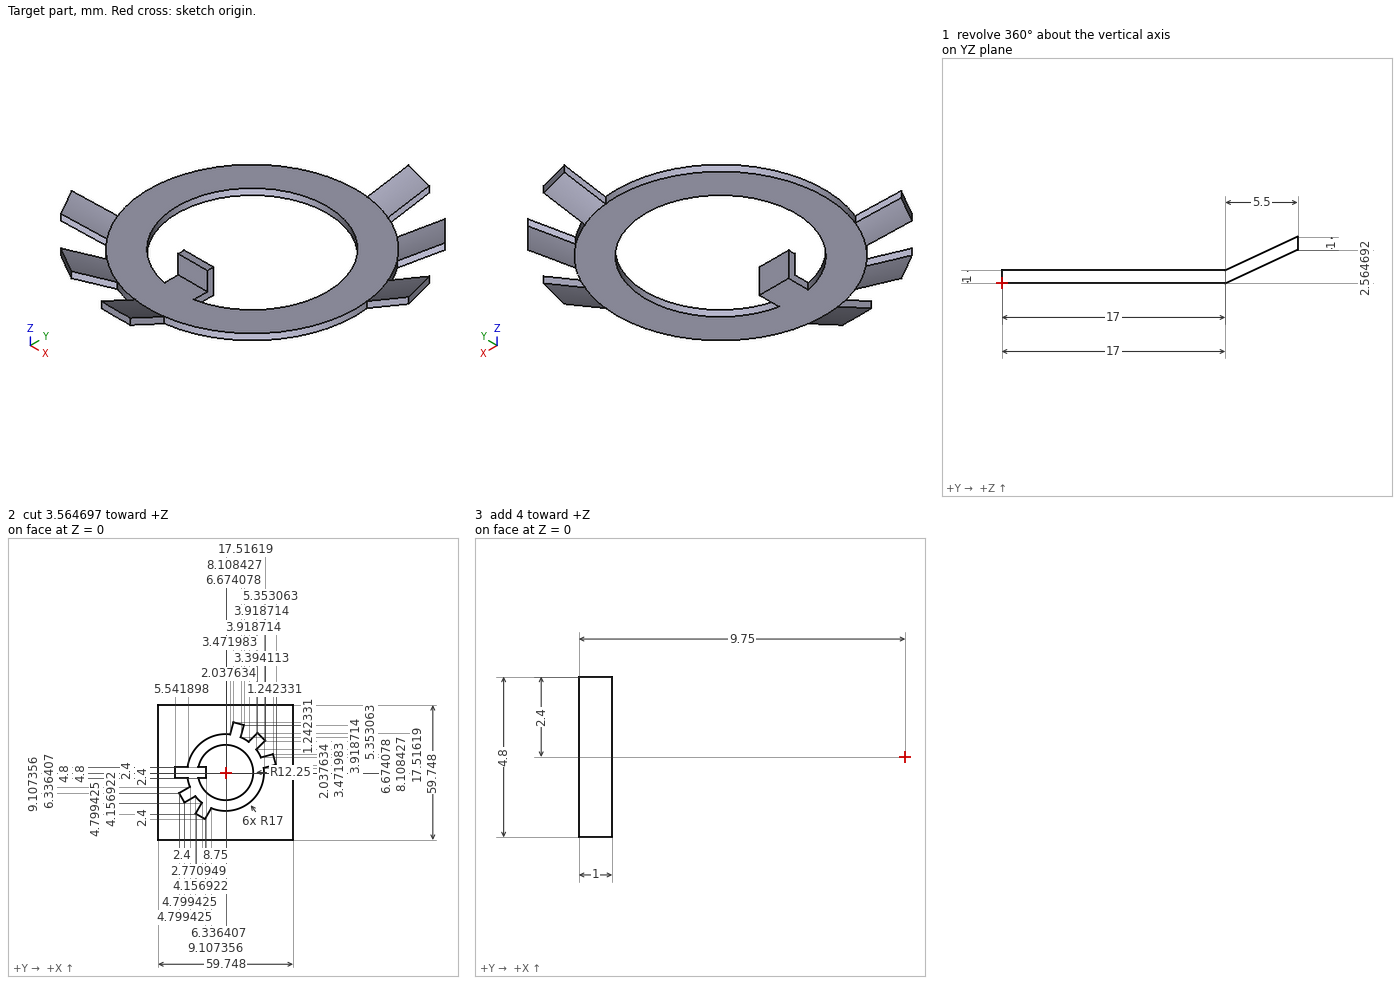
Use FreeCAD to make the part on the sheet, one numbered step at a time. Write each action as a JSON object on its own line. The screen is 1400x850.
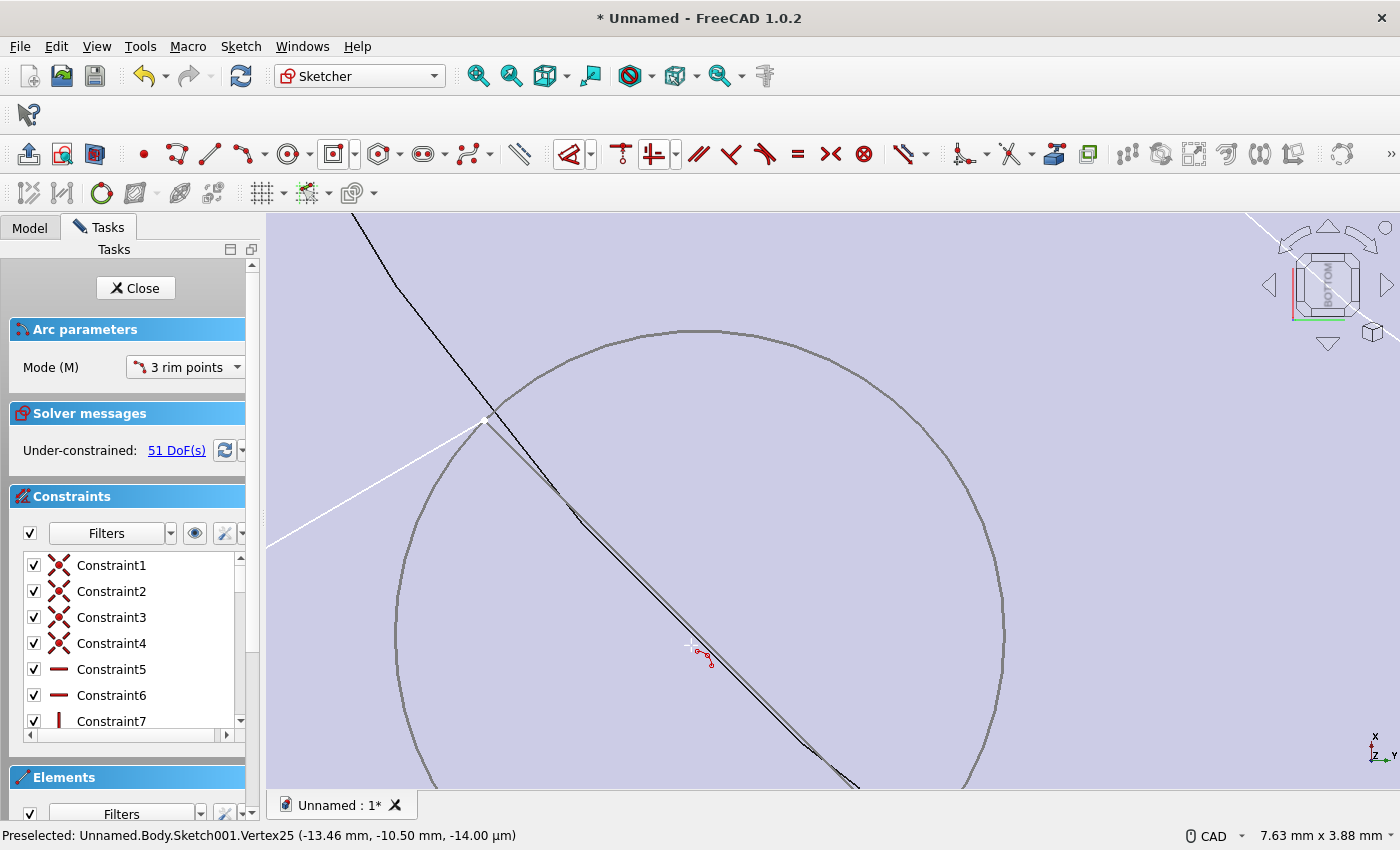
{"action": "left_click", "coordinate": [689, 637]}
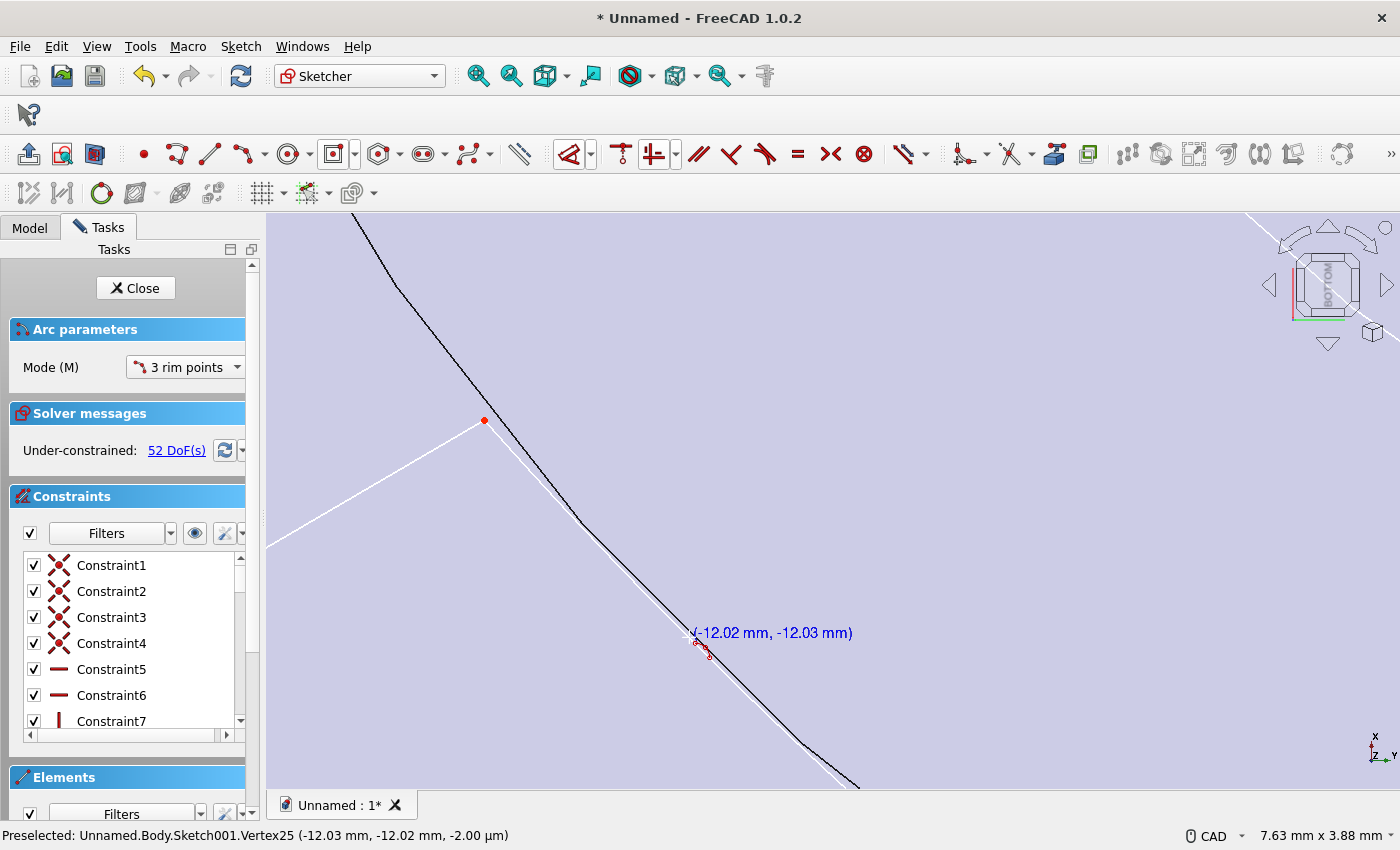
{"action": "scroll", "coordinate": [675, 587], "scroll_direction": "down", "scroll_amount": 15}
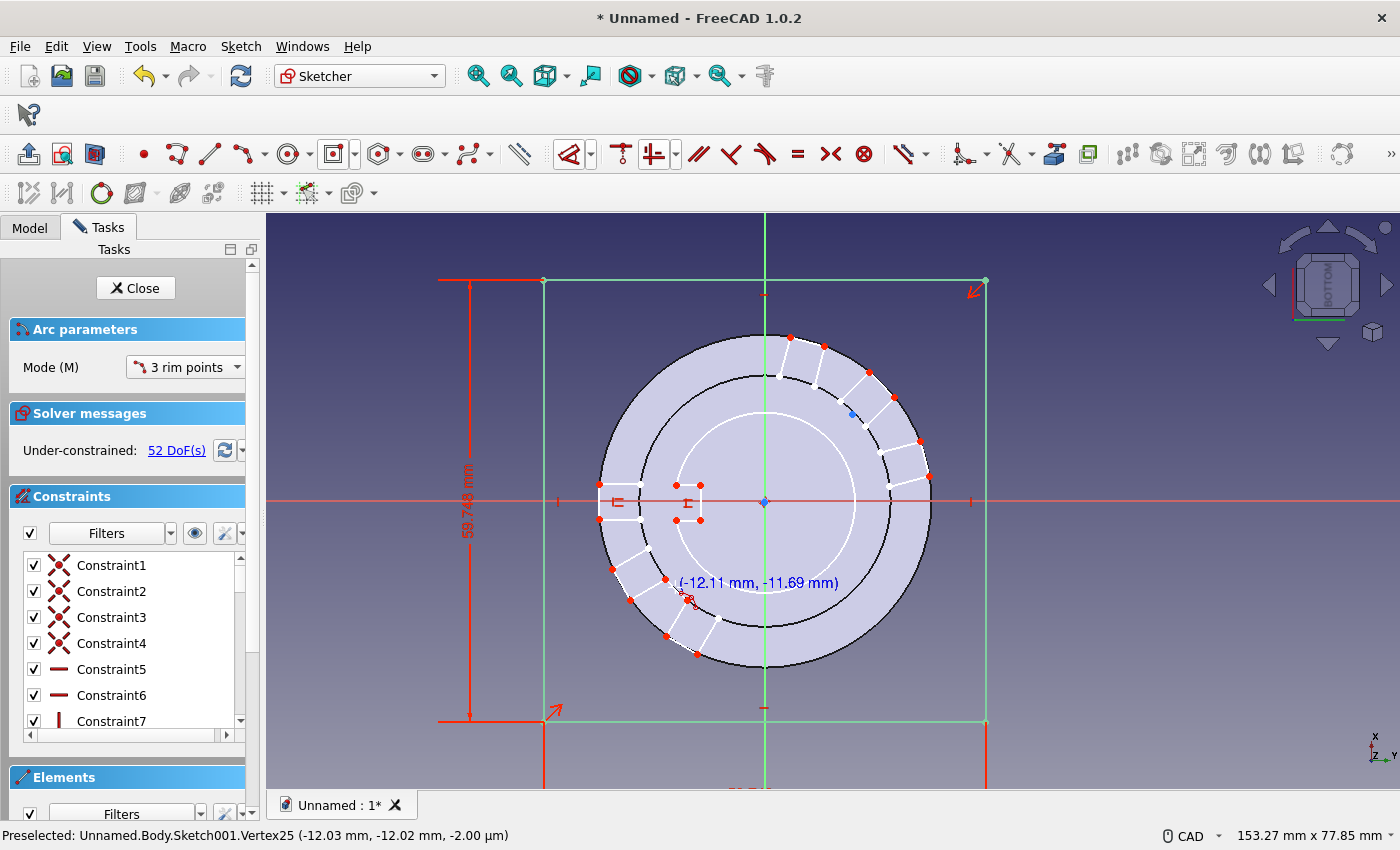
{"action": "left_click", "coordinate": [718, 619]}
{"action": "left_click", "coordinate": [890, 487]}
{"action": "left_click", "coordinate": [842, 601]}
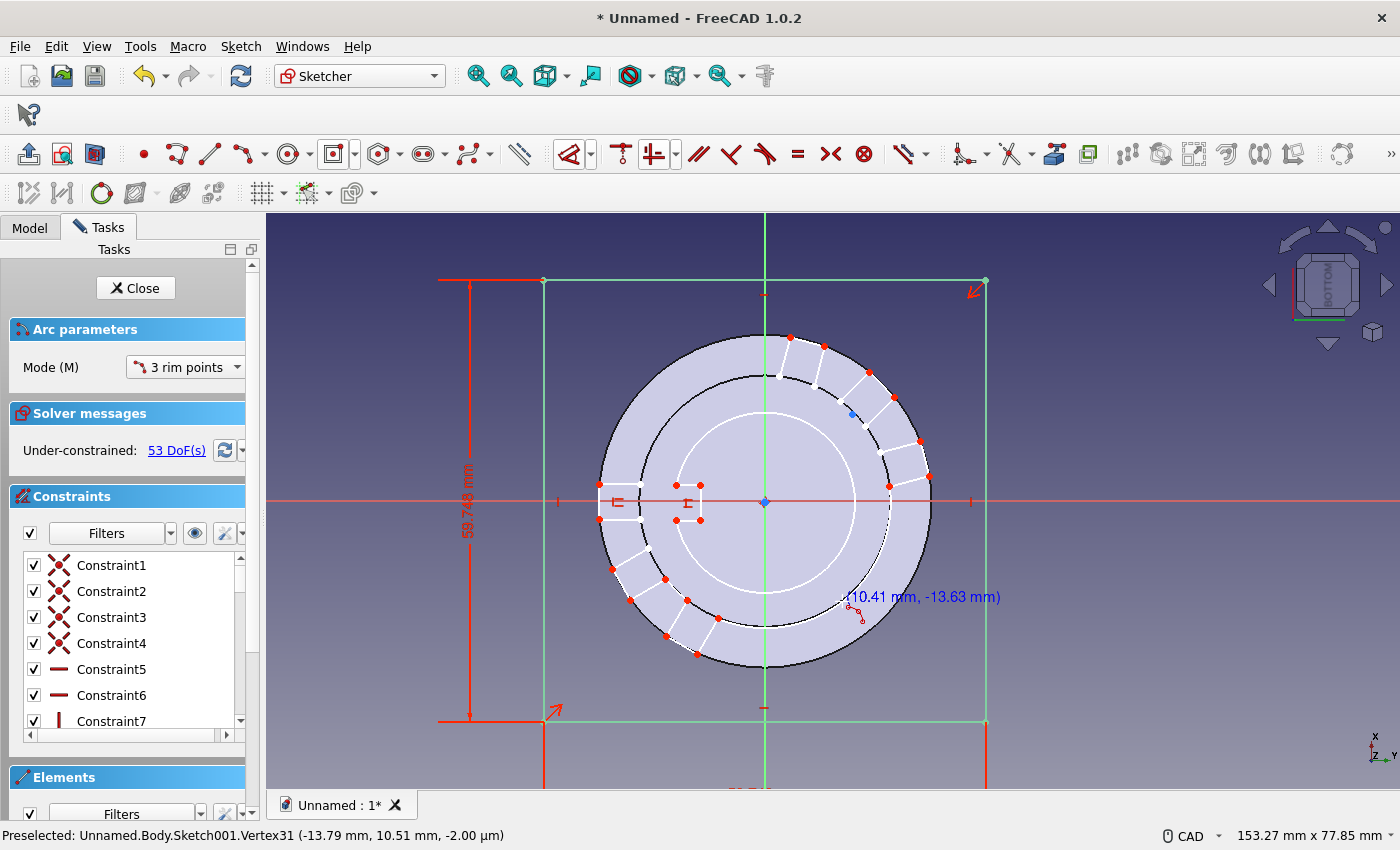
{"action": "left_click", "coordinate": [880, 453]}
{"action": "left_click", "coordinate": [866, 426]}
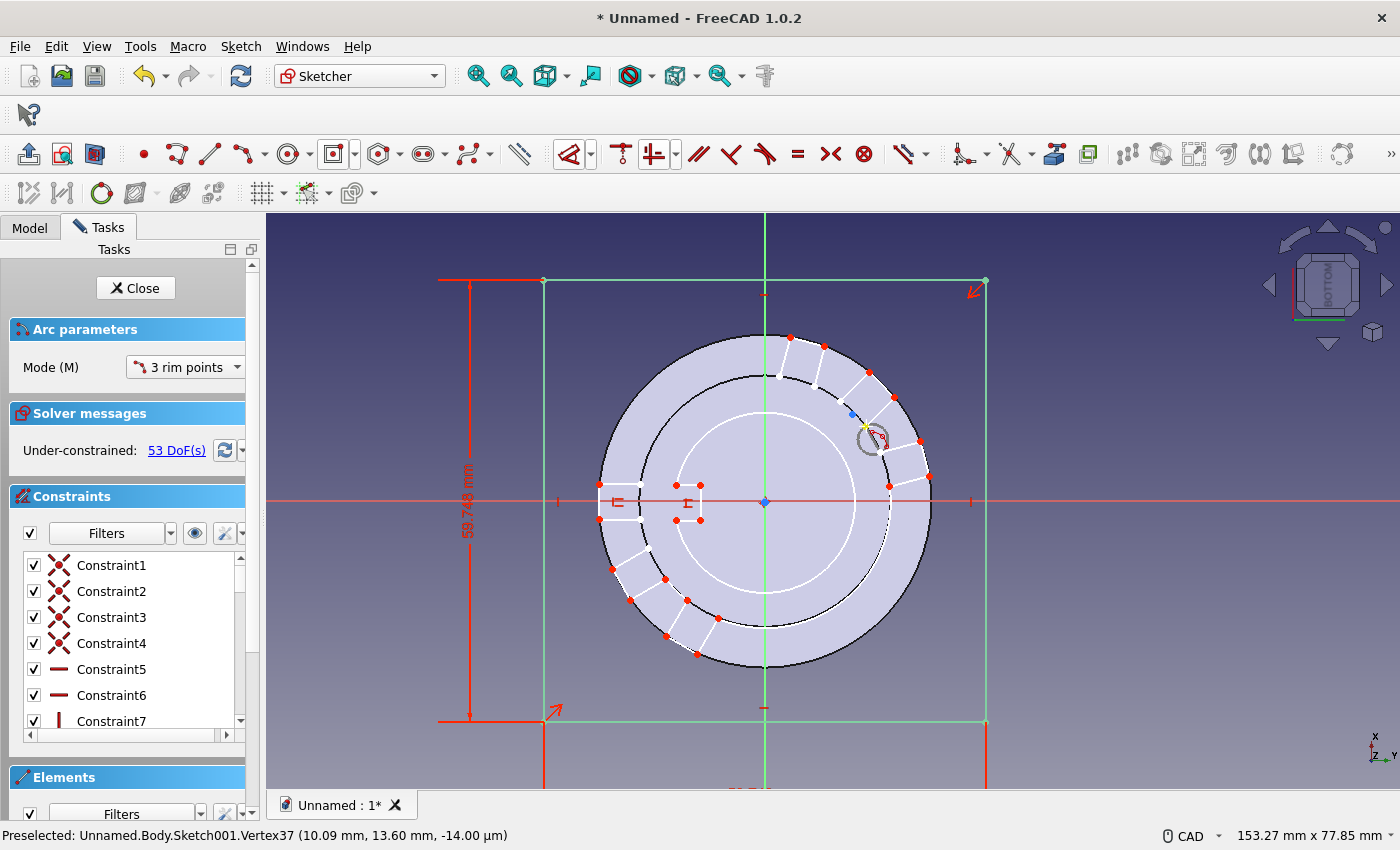
{"action": "scroll", "coordinate": [874, 438], "scroll_direction": "up", "scroll_amount": 15}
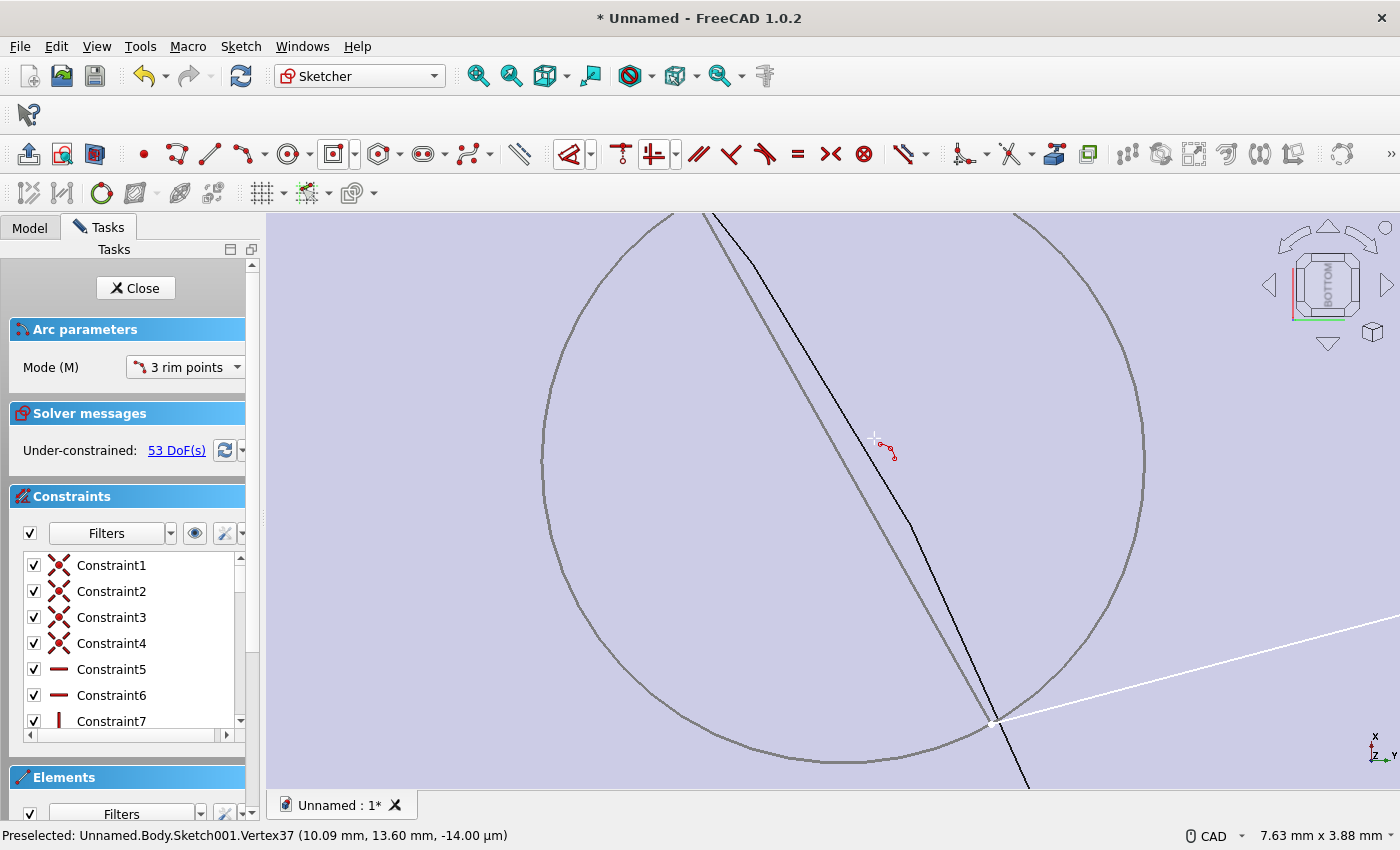
{"action": "left_click", "coordinate": [861, 436]}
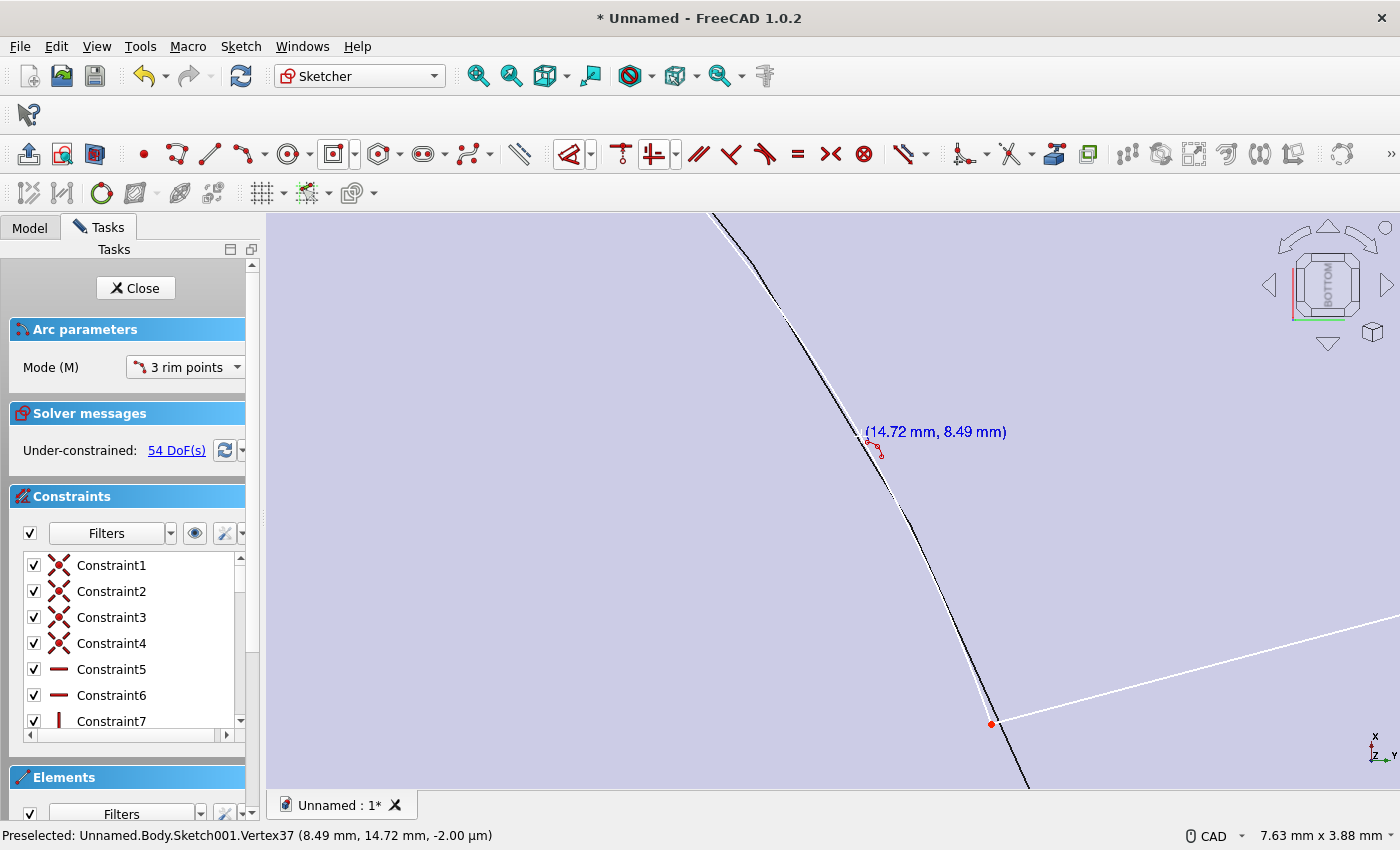
{"action": "scroll", "coordinate": [874, 438], "scroll_direction": "down", "scroll_amount": 15}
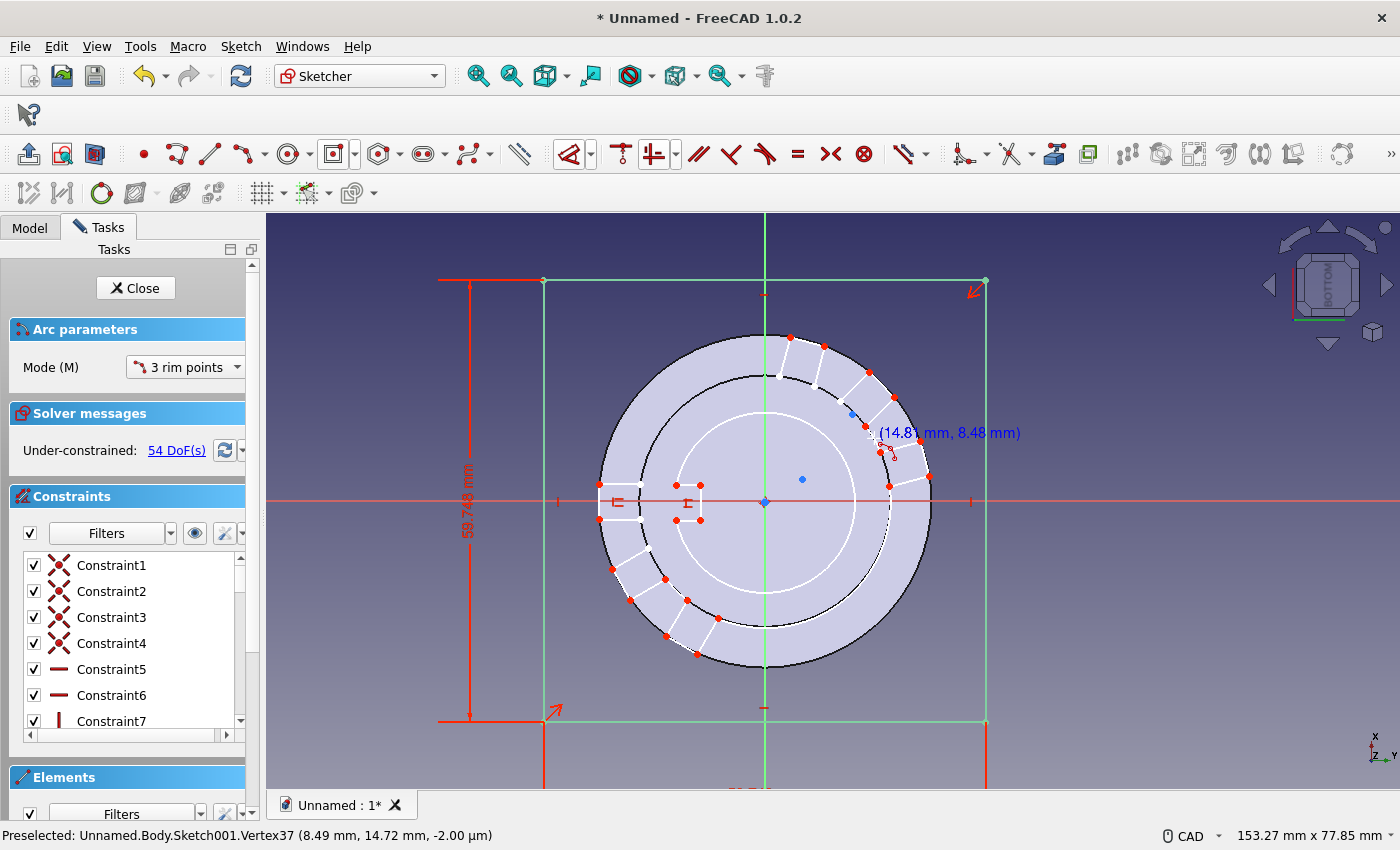
{"action": "left_click", "coordinate": [840, 401]}
{"action": "left_click", "coordinate": [815, 386]}